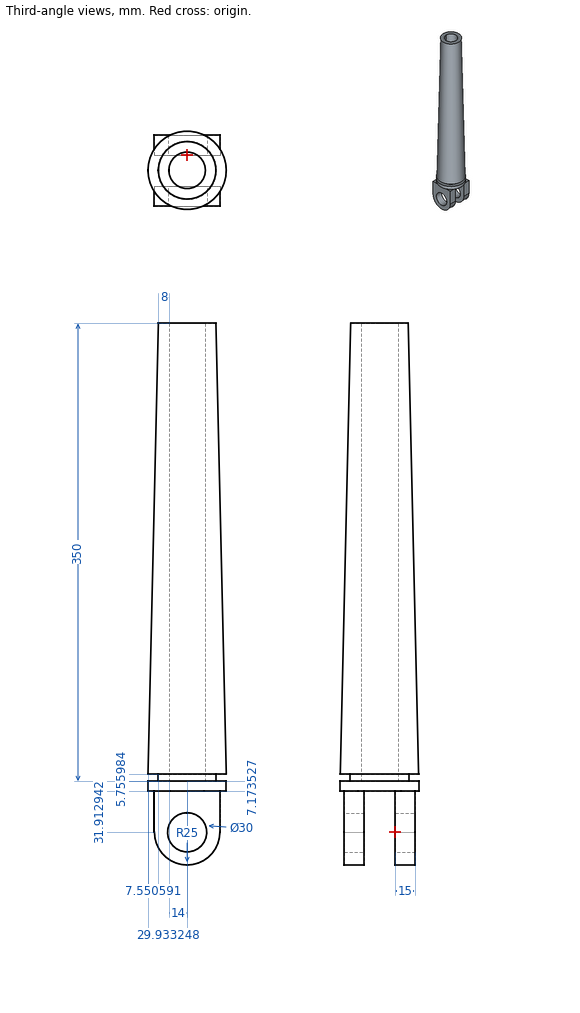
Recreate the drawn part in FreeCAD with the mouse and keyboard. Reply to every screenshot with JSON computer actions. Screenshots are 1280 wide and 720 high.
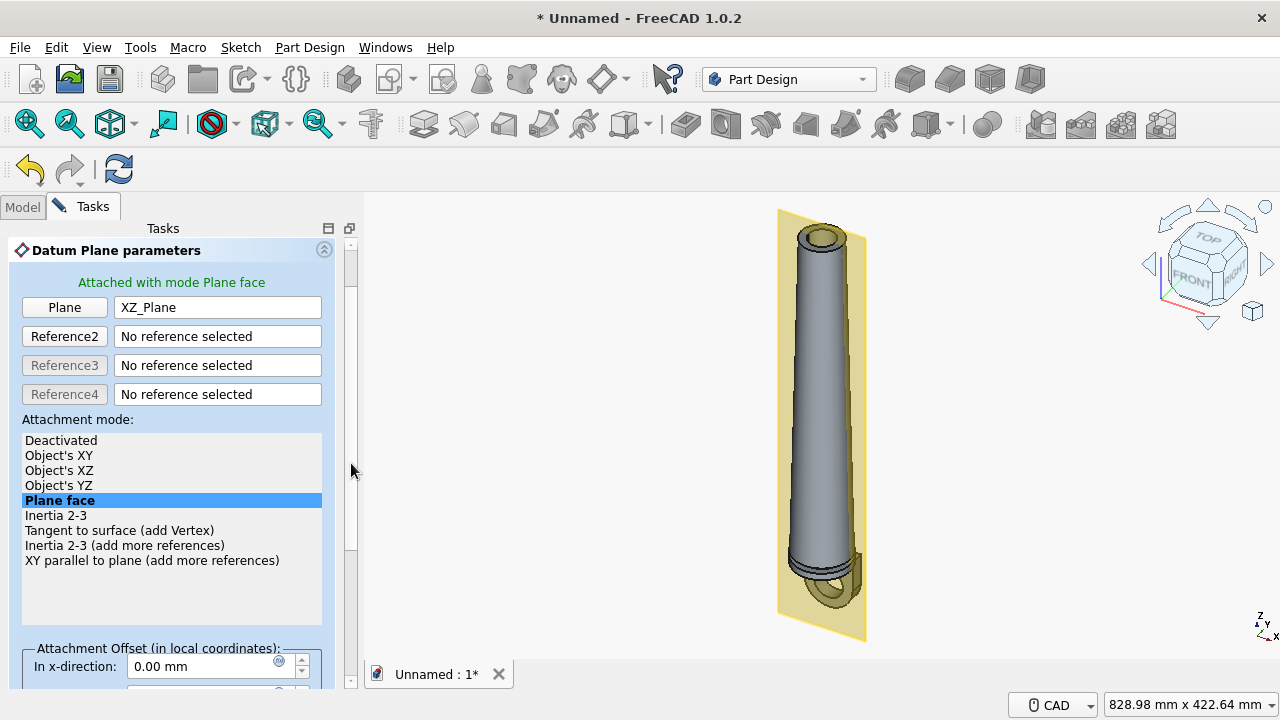
{"action": "left_click", "coordinate": [124, 267]}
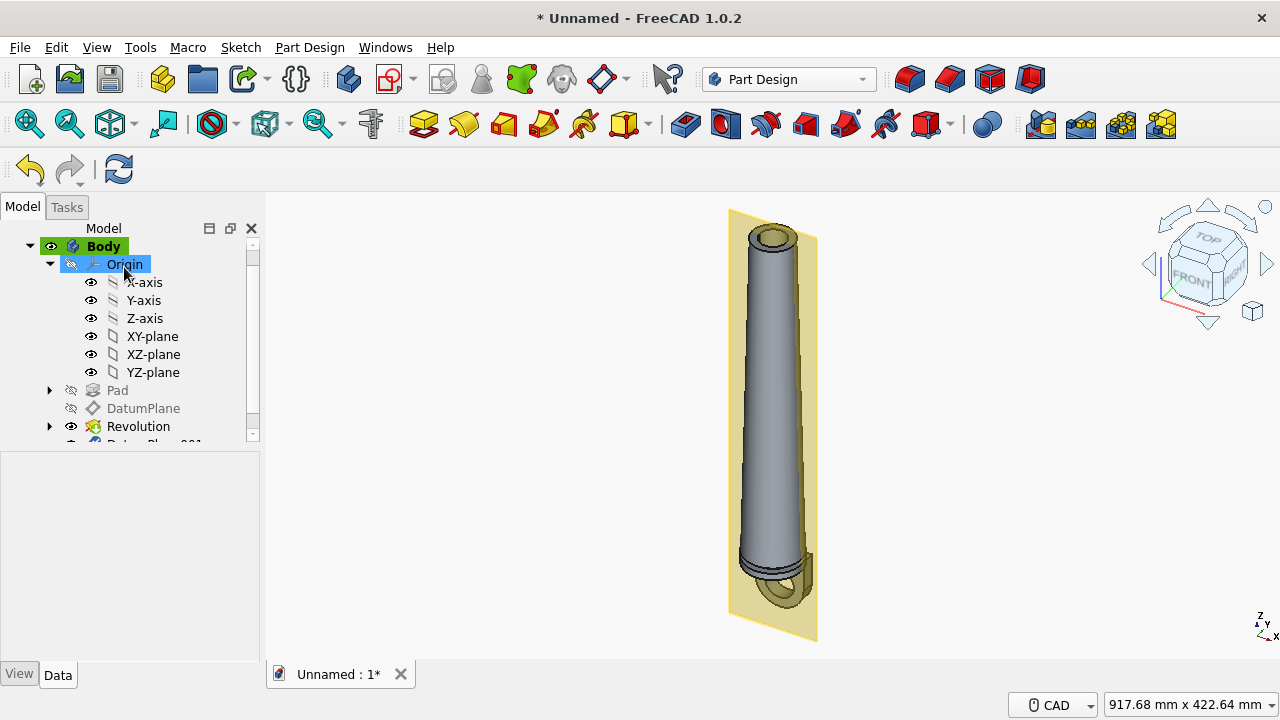
{"action": "left_click", "coordinate": [116, 390]}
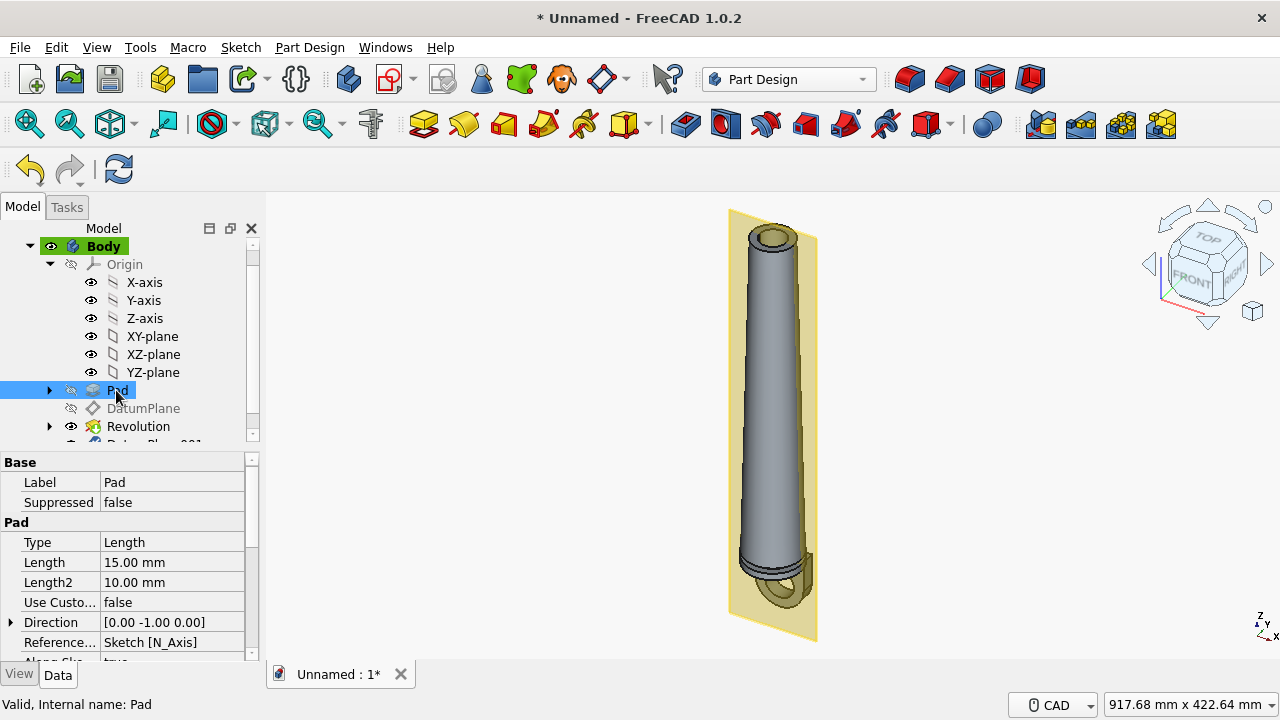
{"action": "left_click", "coordinate": [1042, 124]}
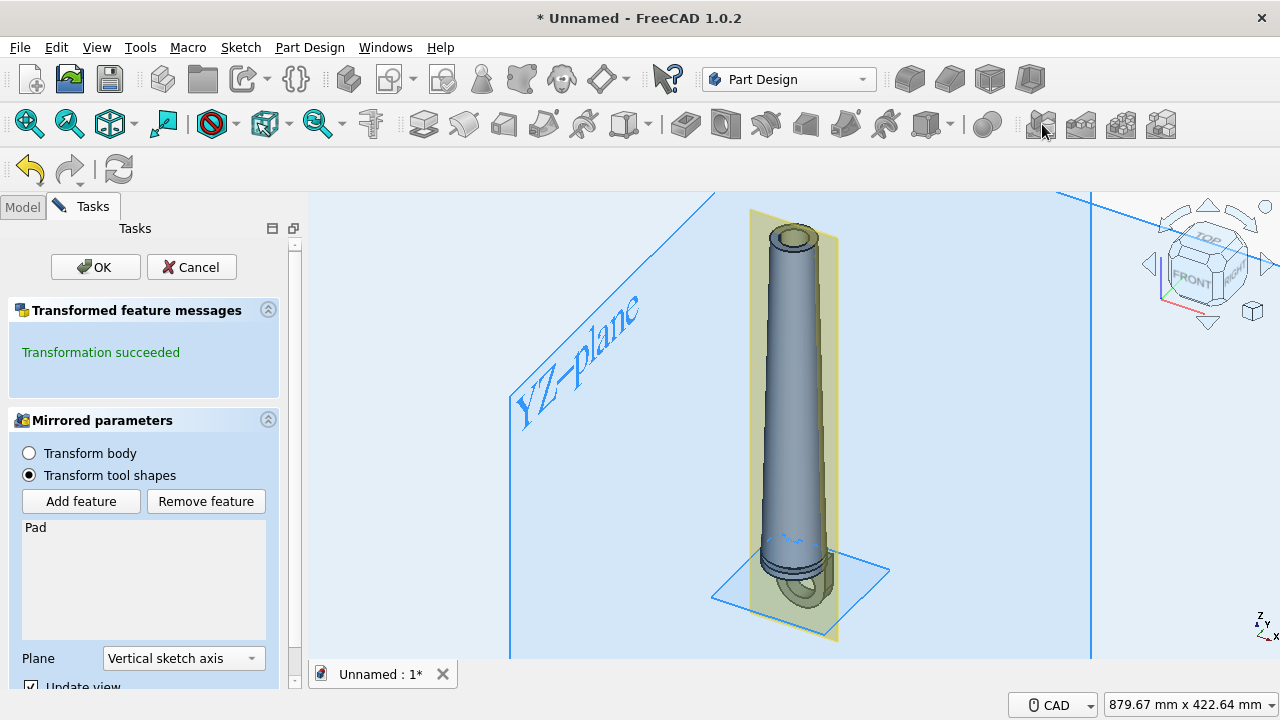
{"action": "left_click", "coordinate": [184, 658]}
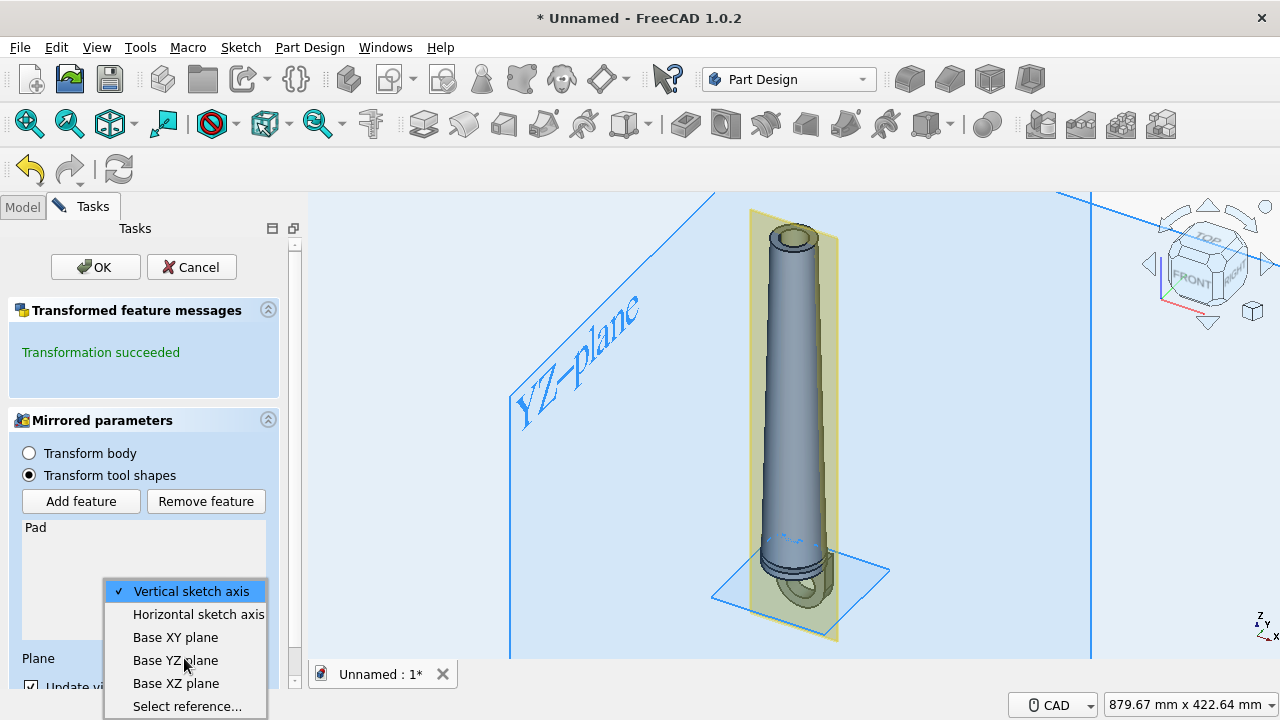
{"action": "left_click", "coordinate": [184, 706]}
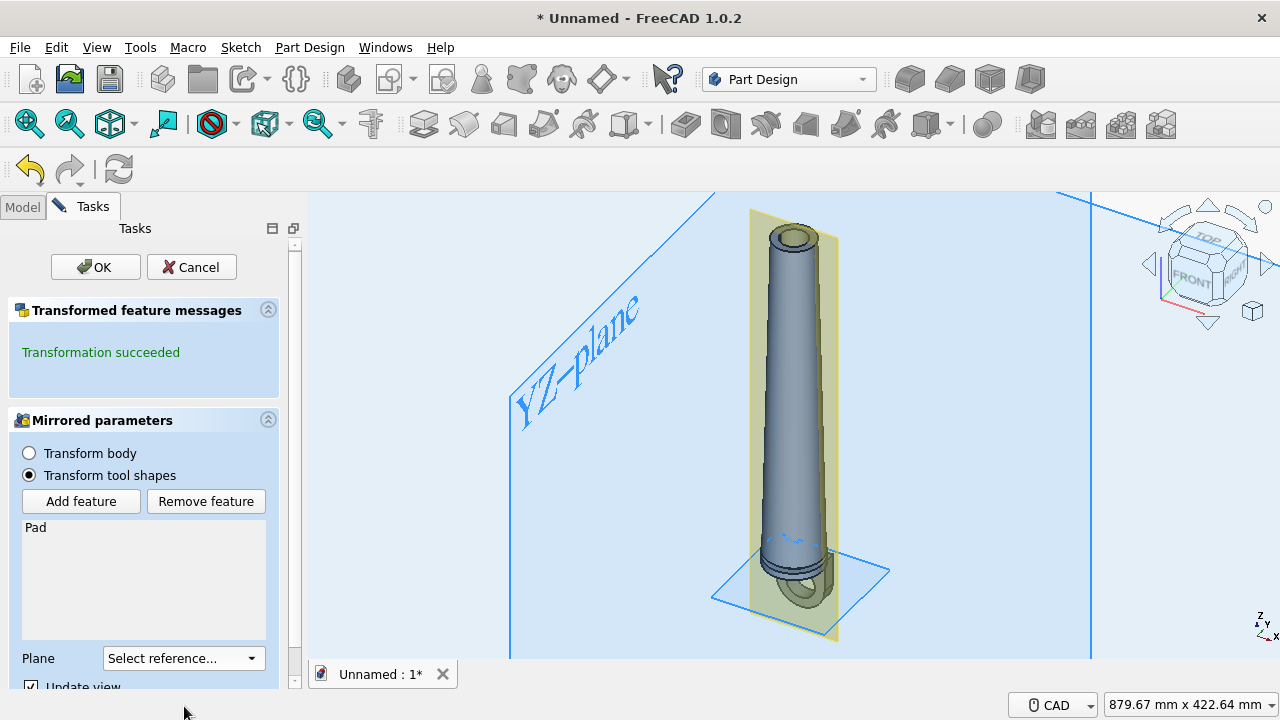
{"action": "left_click", "coordinate": [23, 206]}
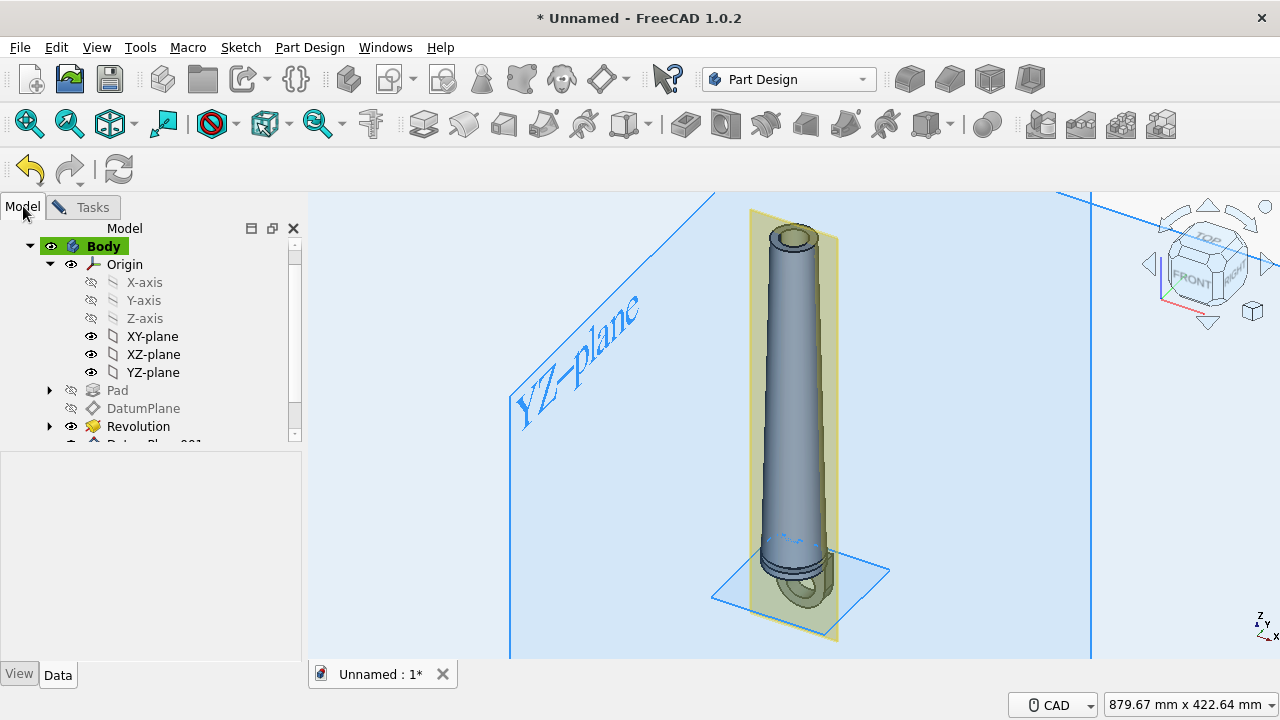
{"action": "scroll", "coordinate": [120, 332], "scroll_direction": "down", "scroll_amount": 3}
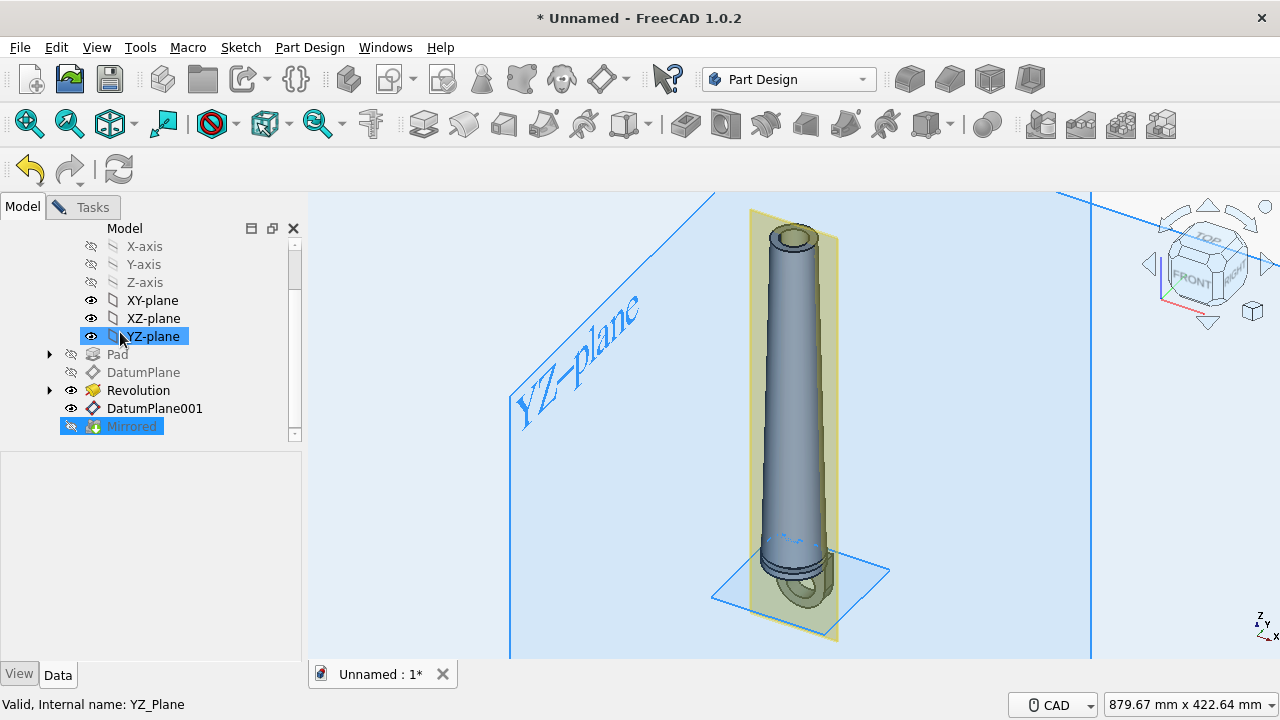
{"action": "left_click", "coordinate": [116, 408]}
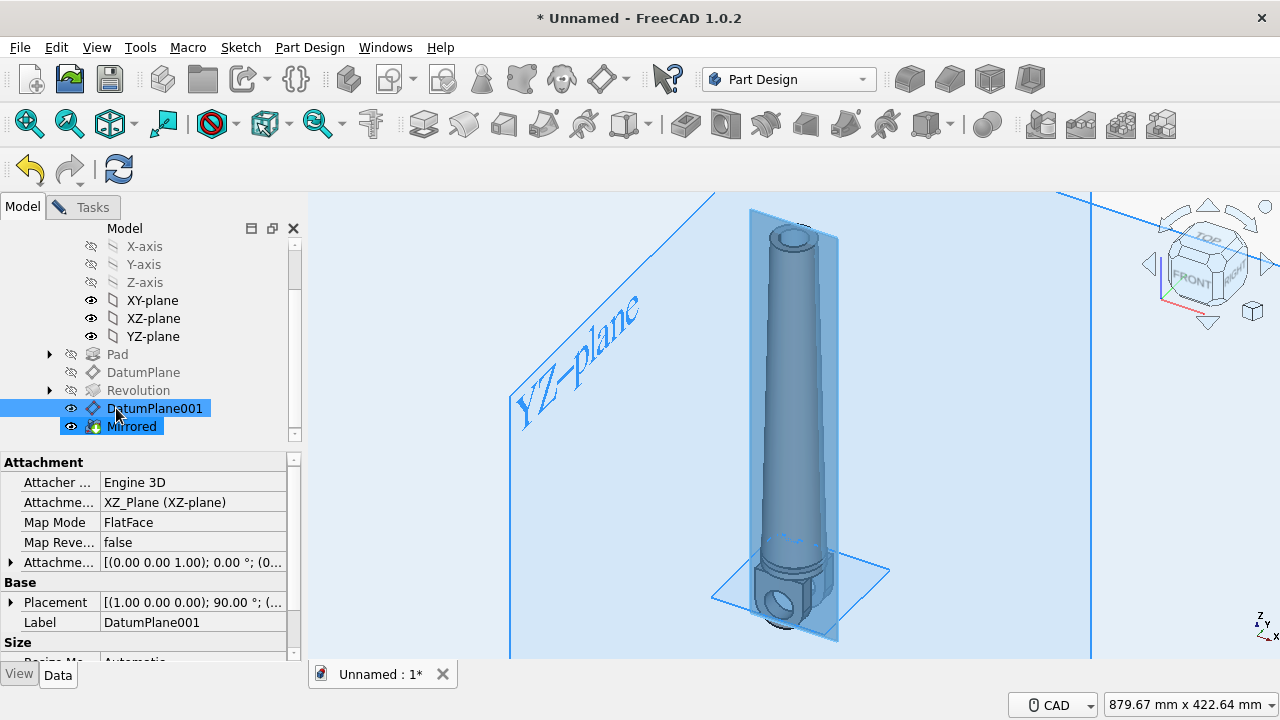
{"action": "left_click", "coordinate": [84, 206]}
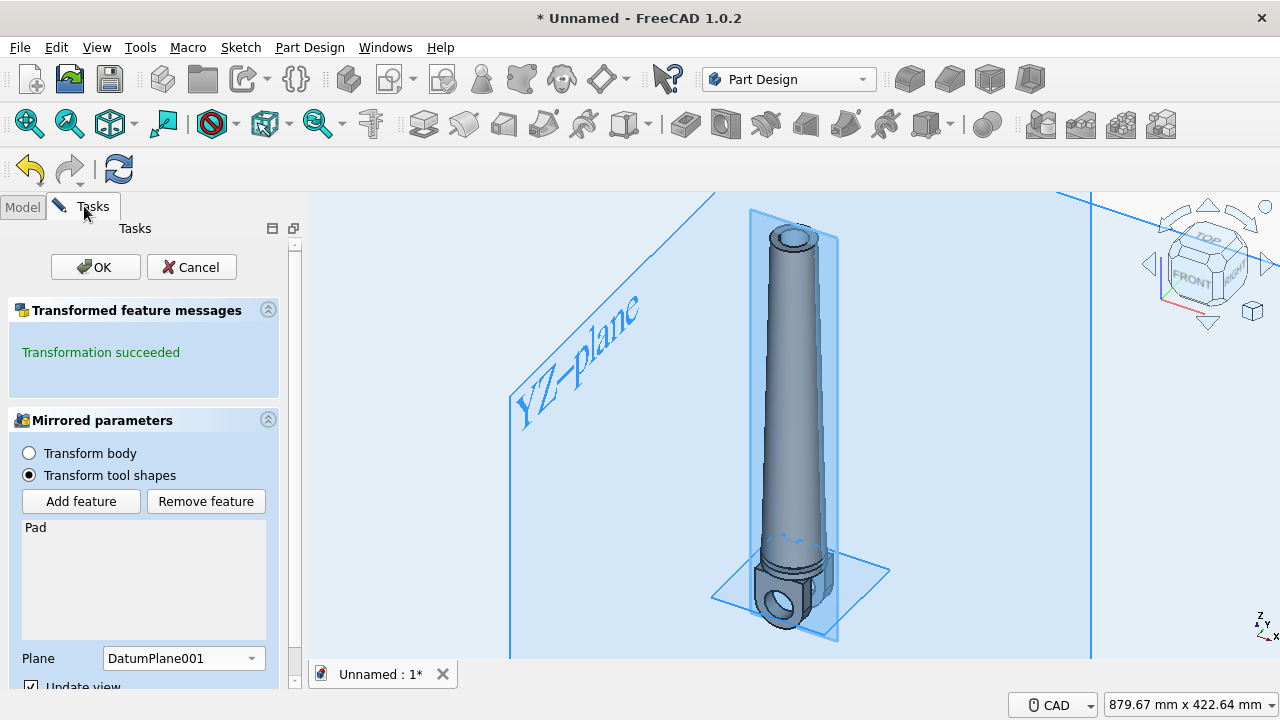
{"action": "left_click", "coordinate": [96, 267]}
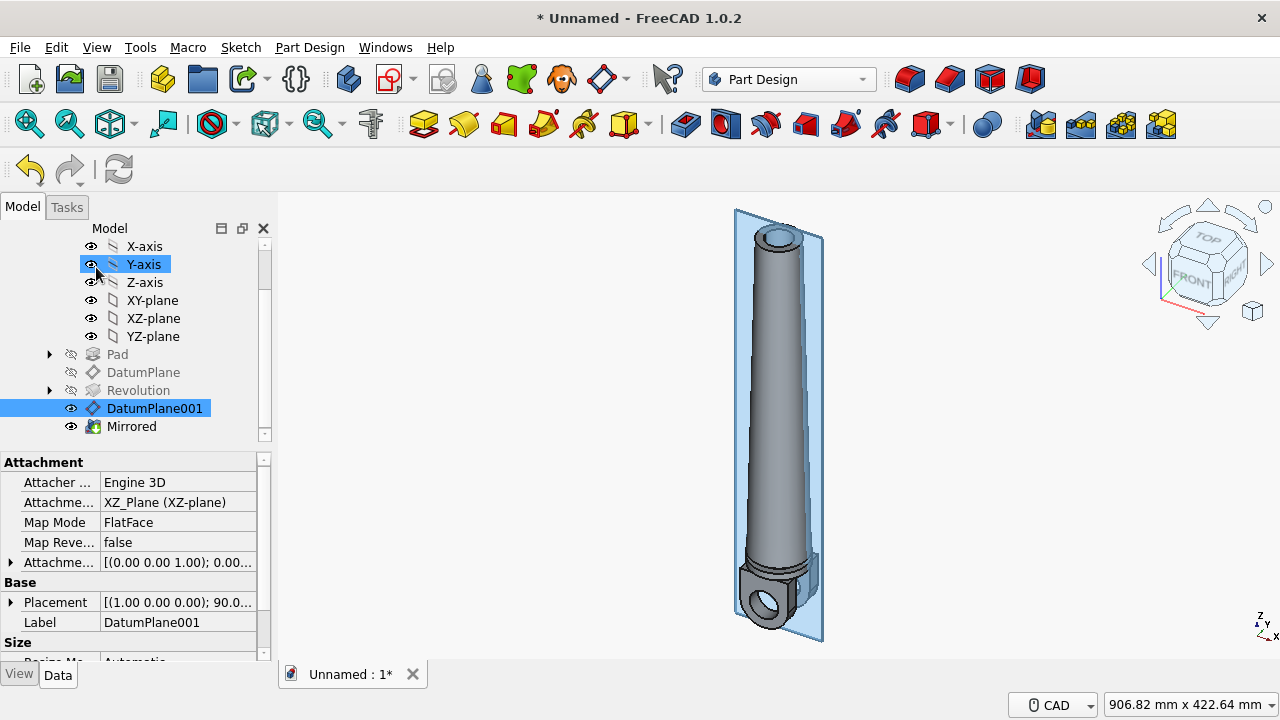
{"action": "left_click", "coordinate": [116, 408]}
{"action": "key", "text": "space"}